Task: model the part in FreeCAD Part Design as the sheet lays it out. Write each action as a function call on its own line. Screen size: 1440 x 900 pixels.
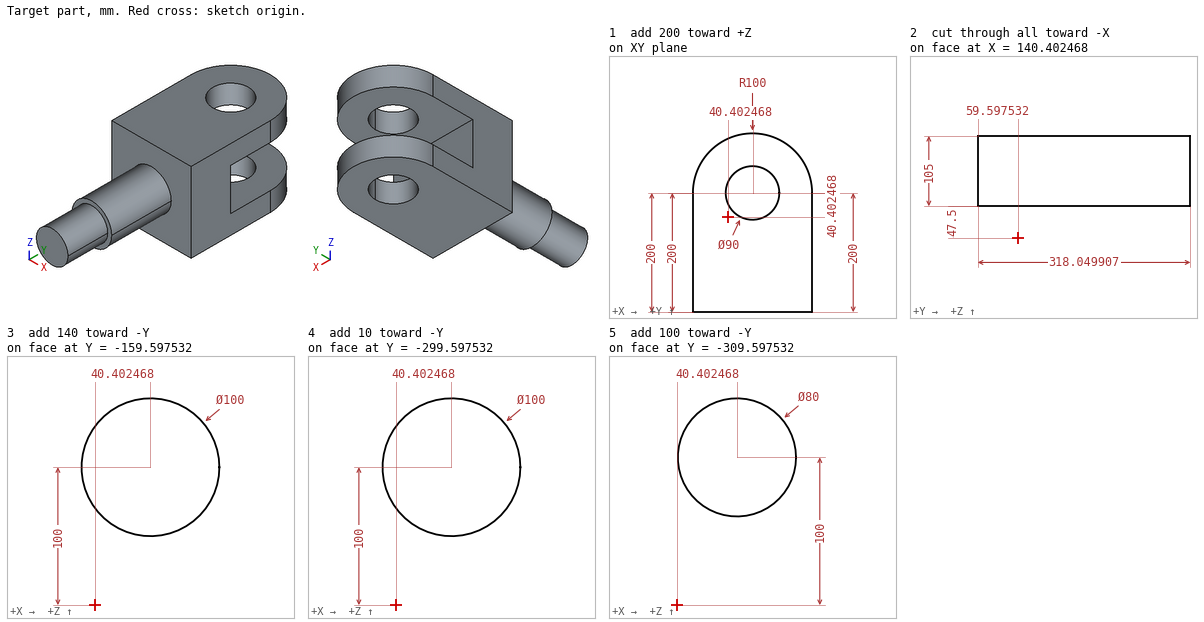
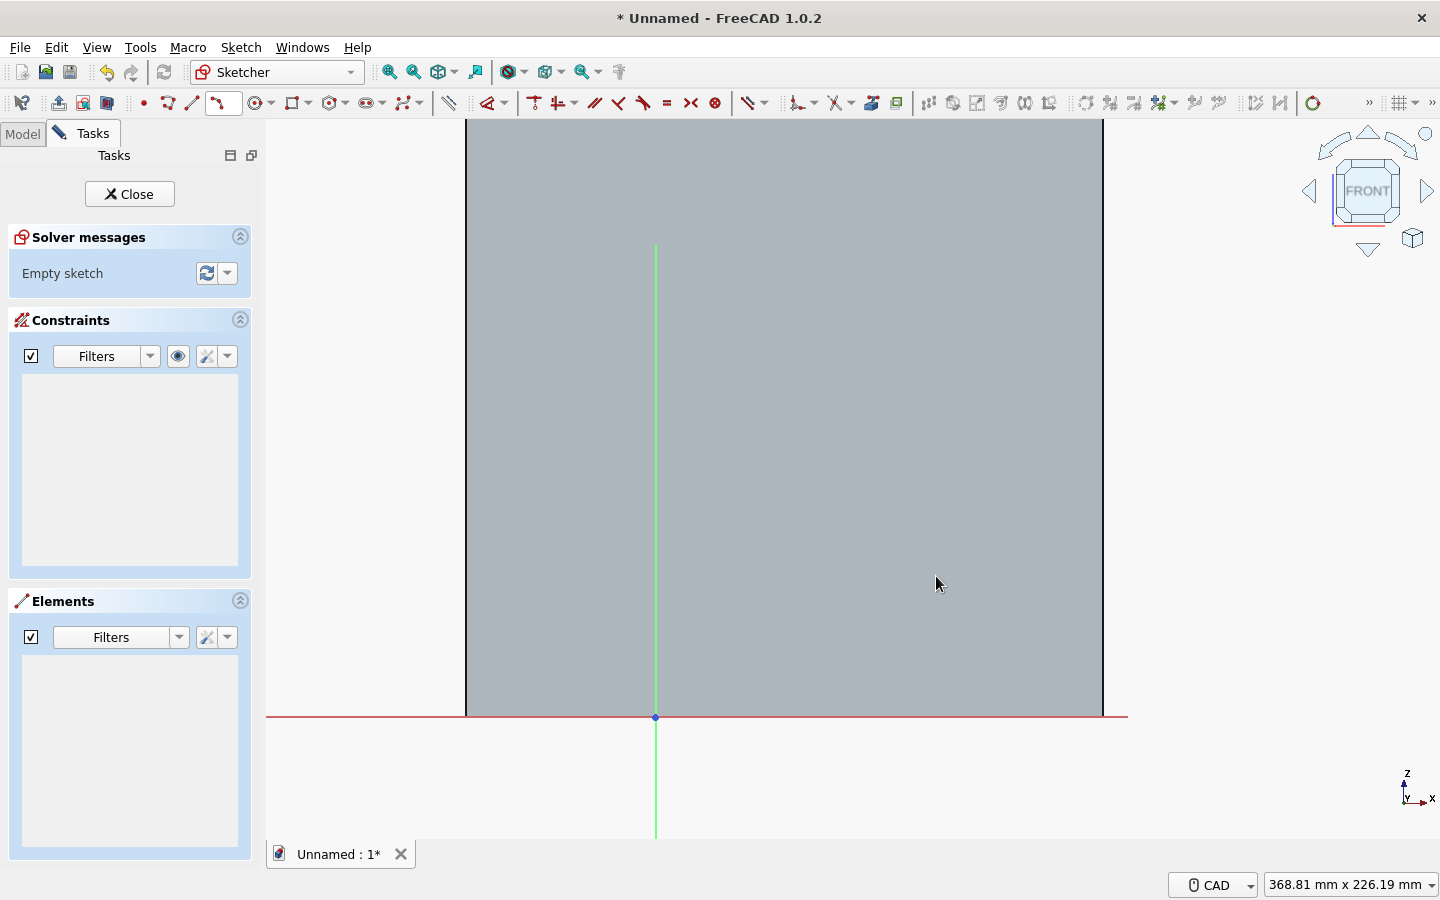
key(g)
key(c)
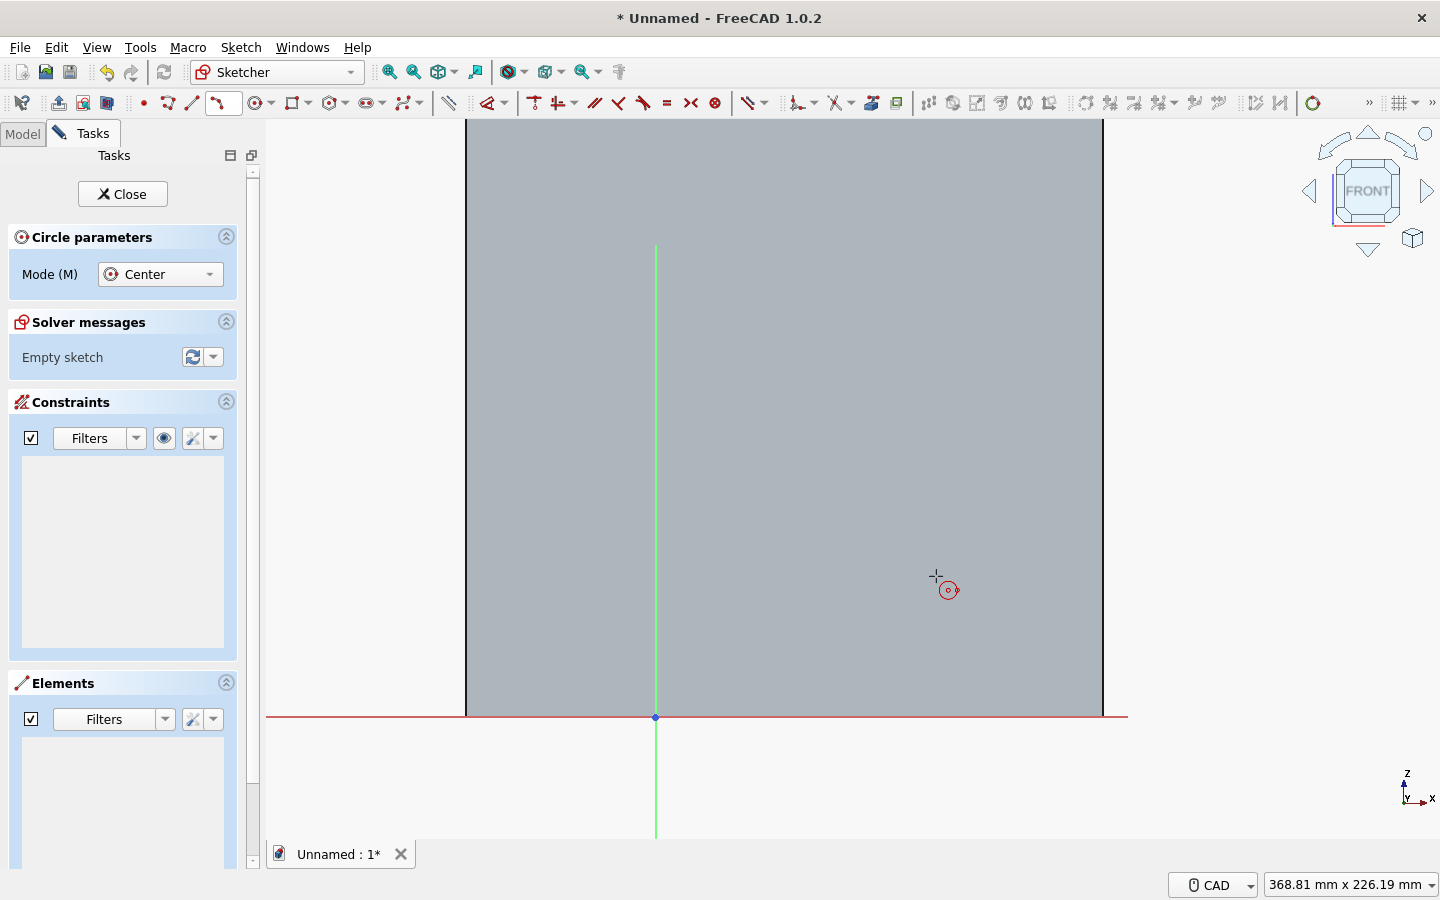
click(784, 399)
click(897, 286)
key(Escape)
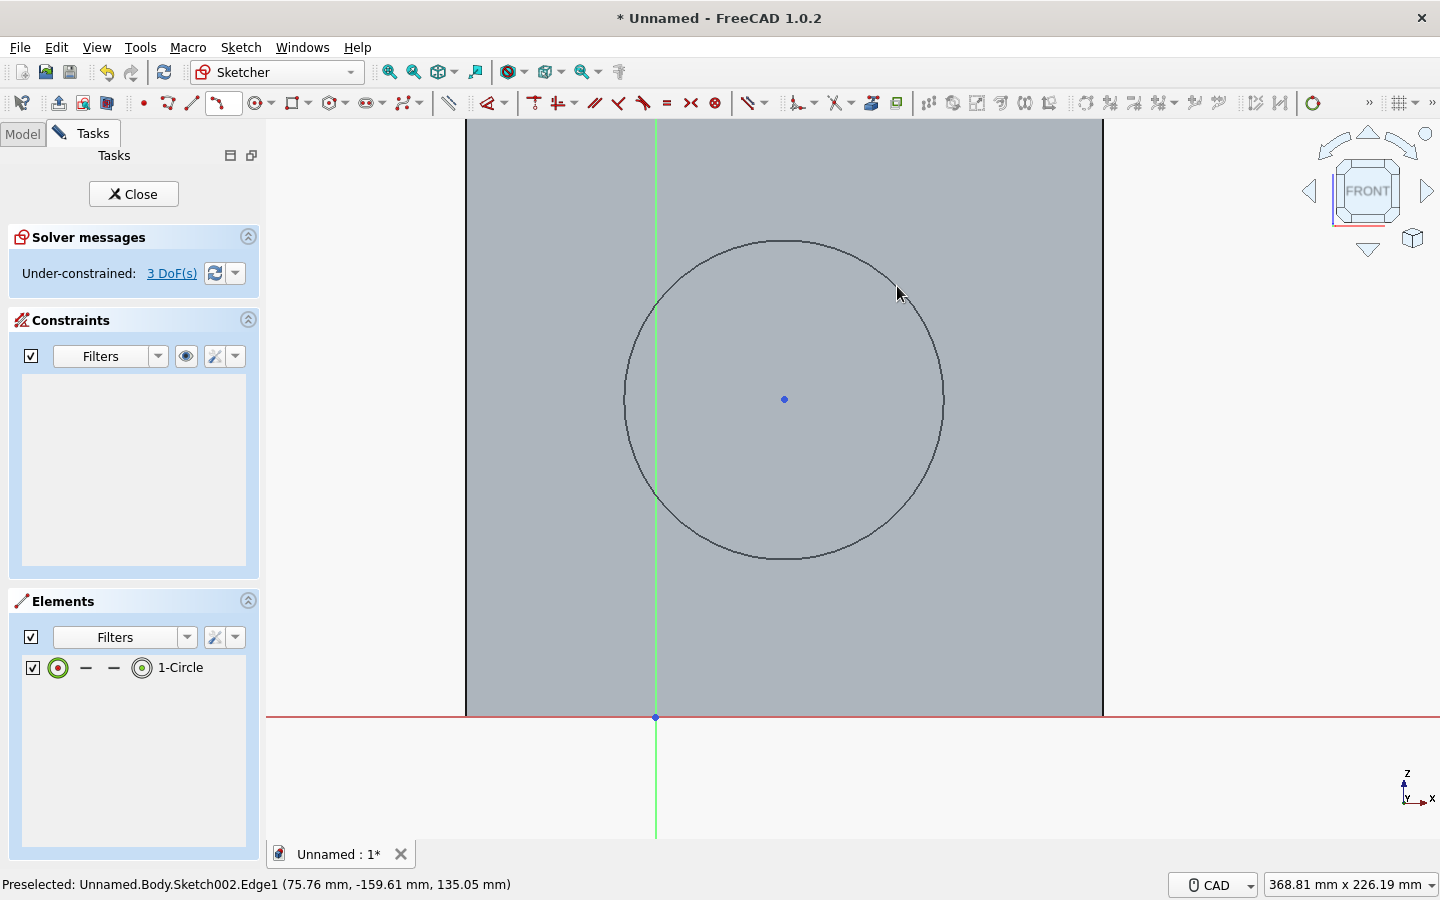
click(488, 104)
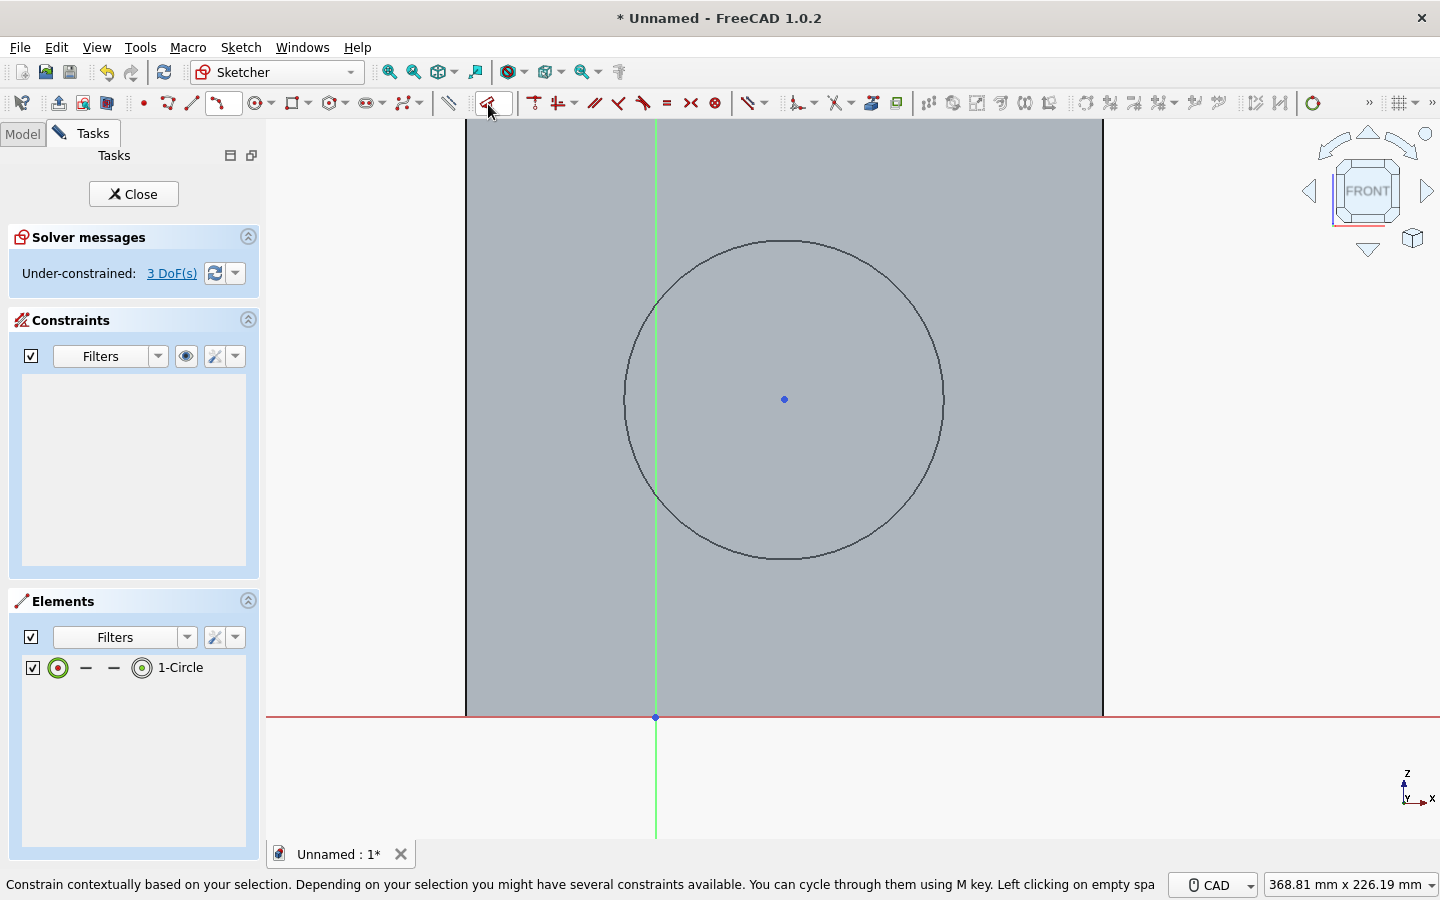
click(897, 287)
click(920, 264)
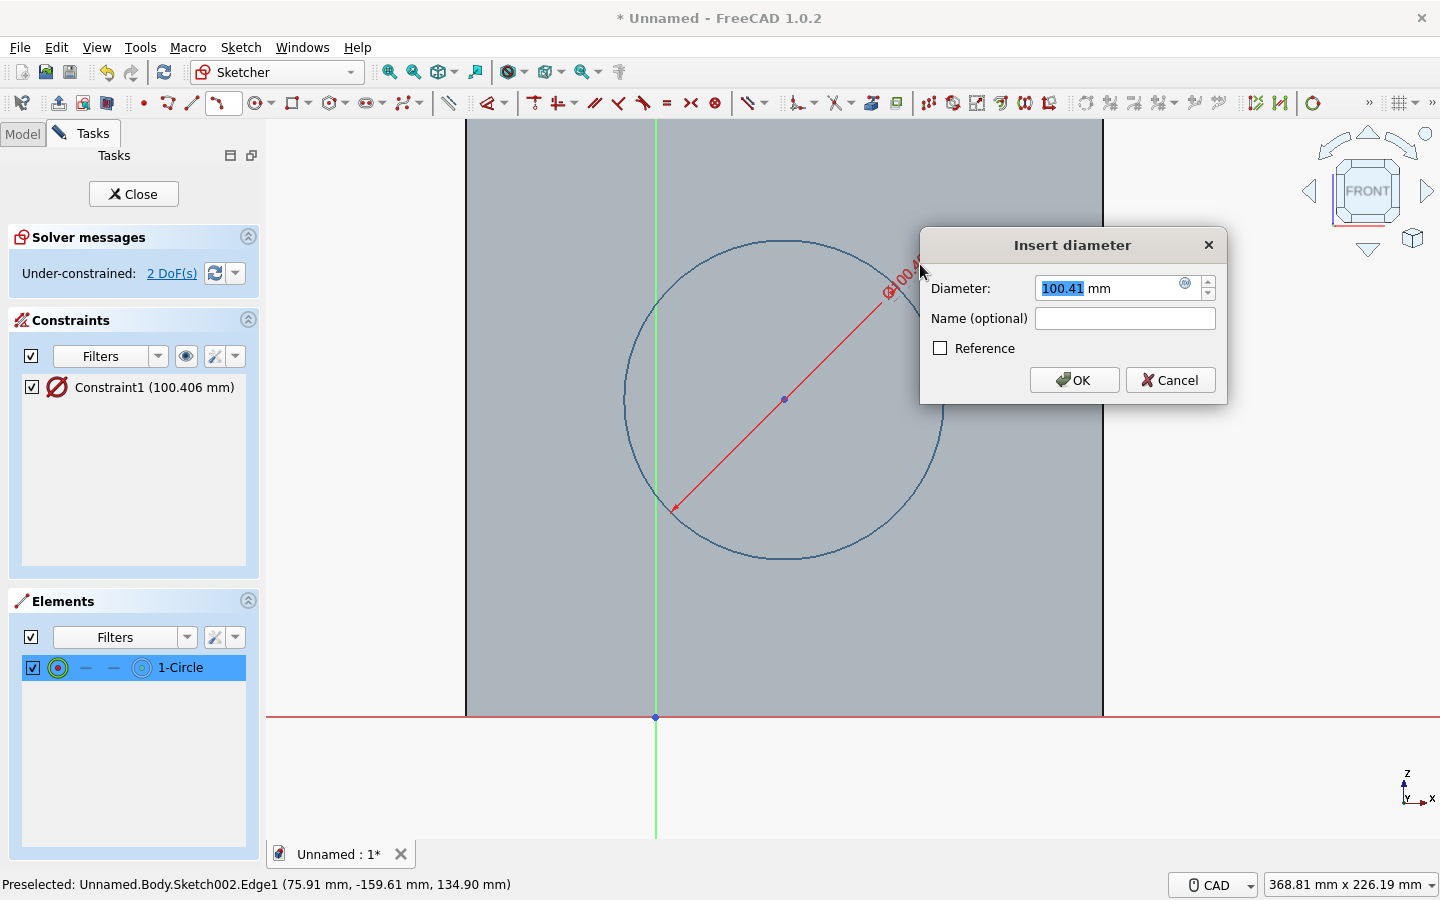
text(100)
key(Return)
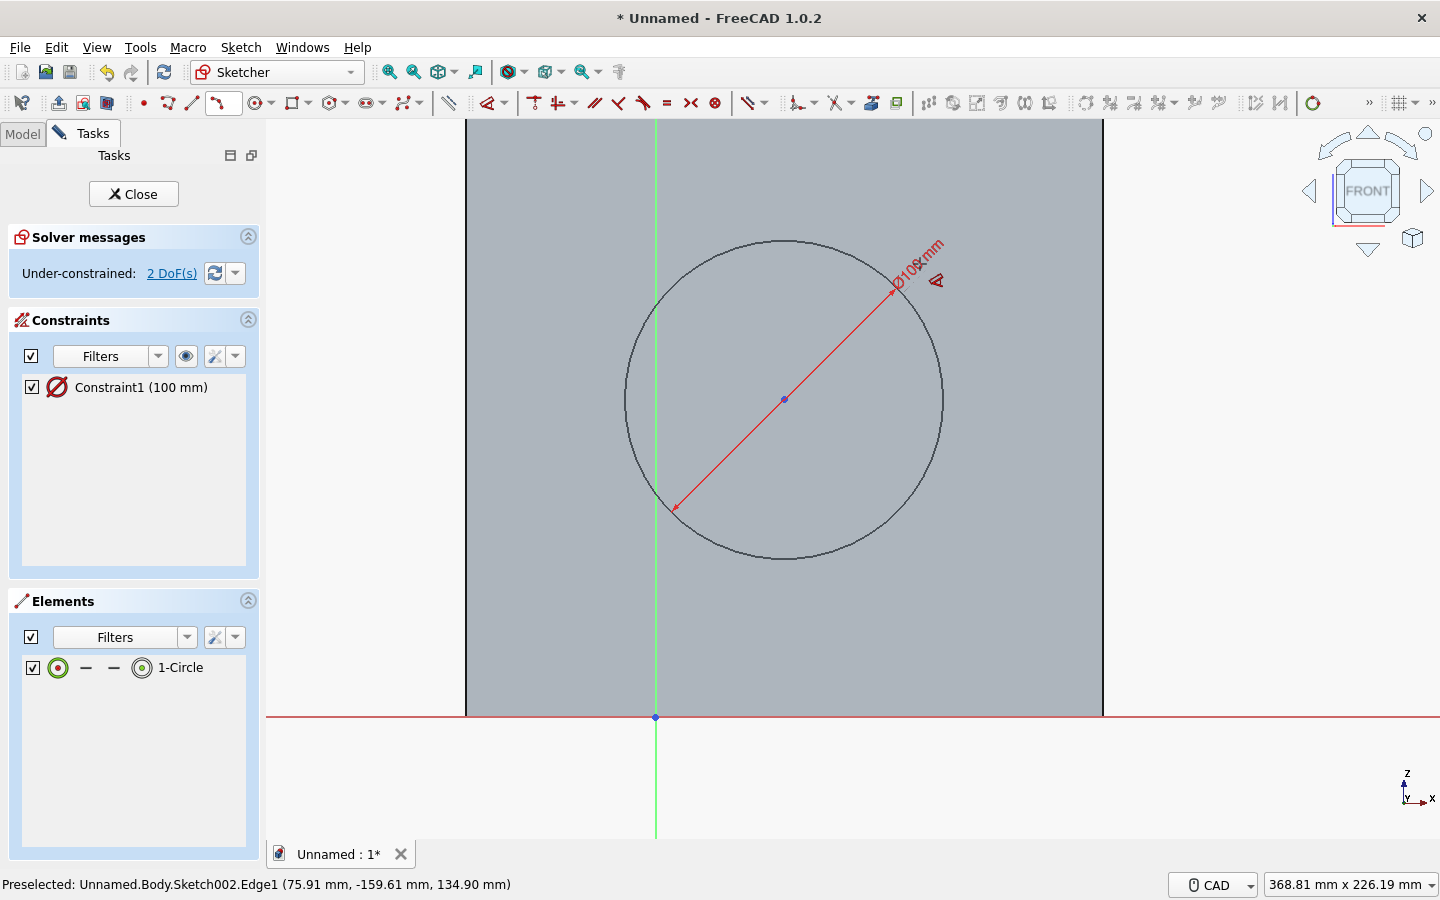
click(784, 400)
click(622, 559)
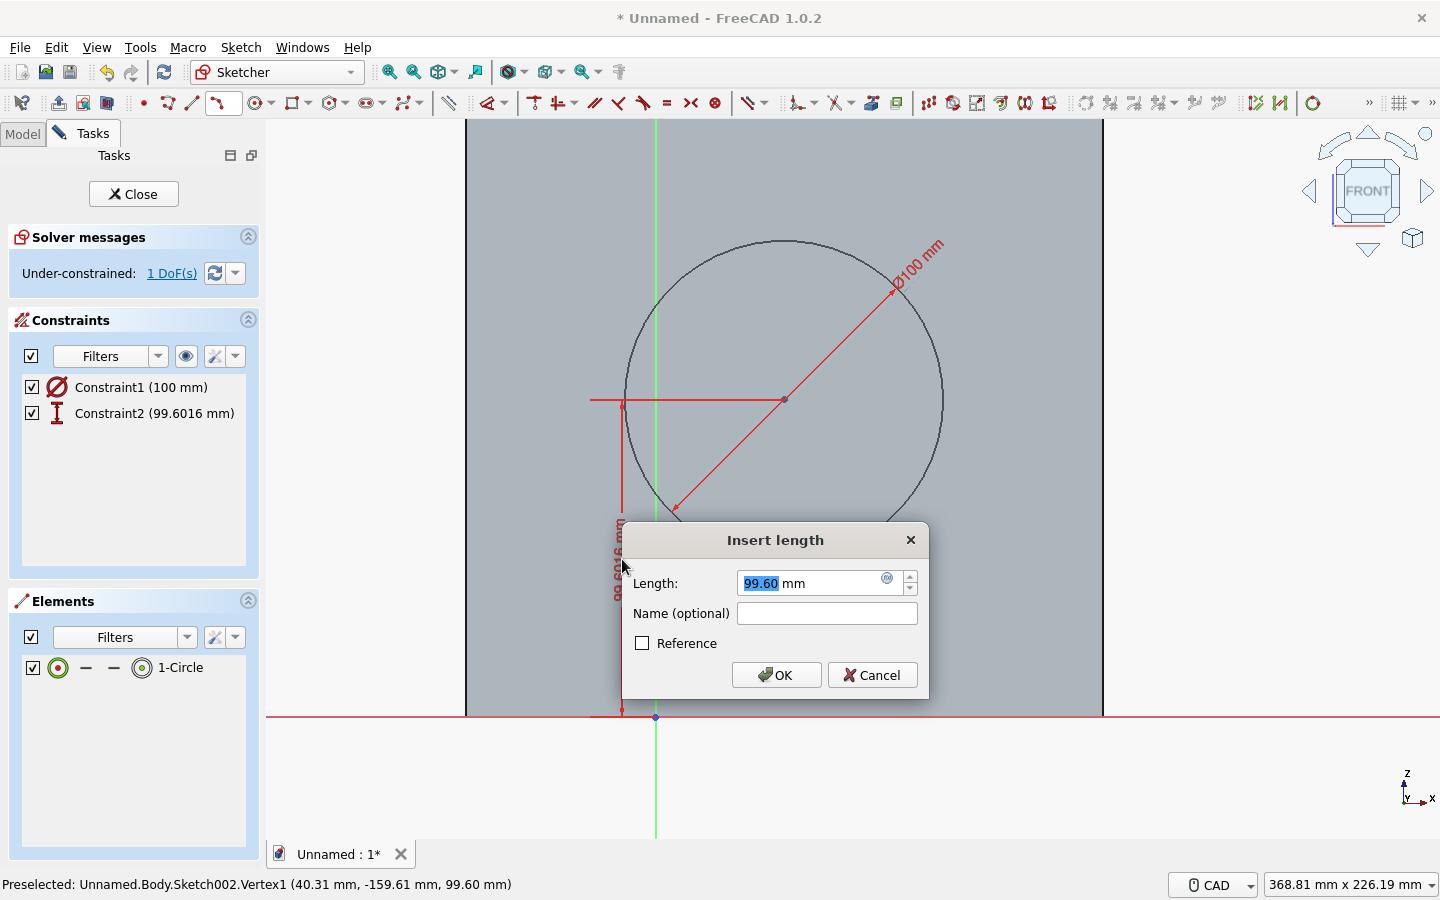
text(100)
key(Return)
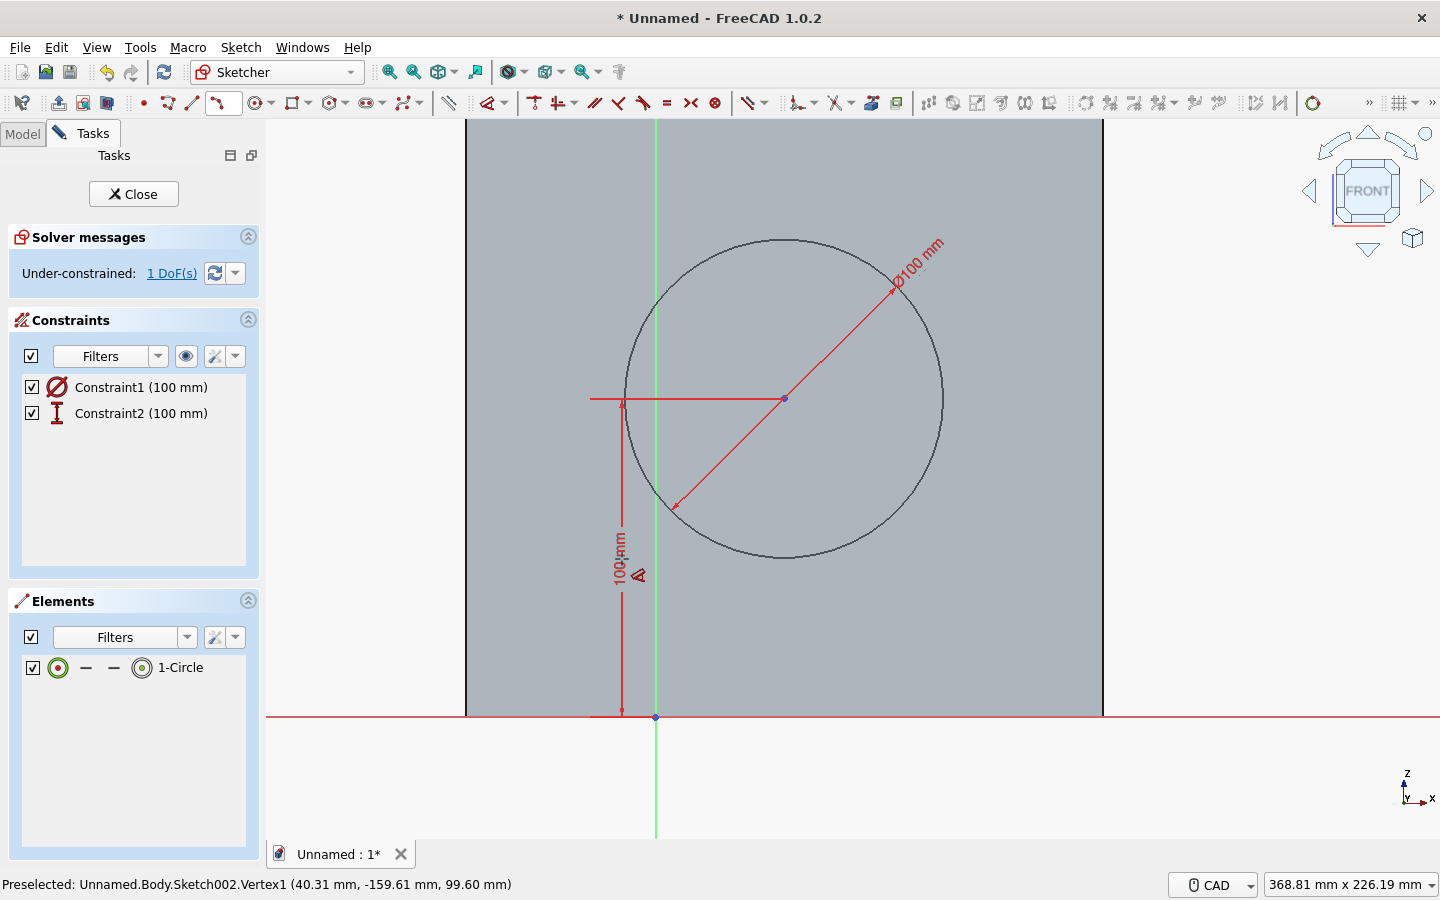
click(784, 399)
click(720, 751)